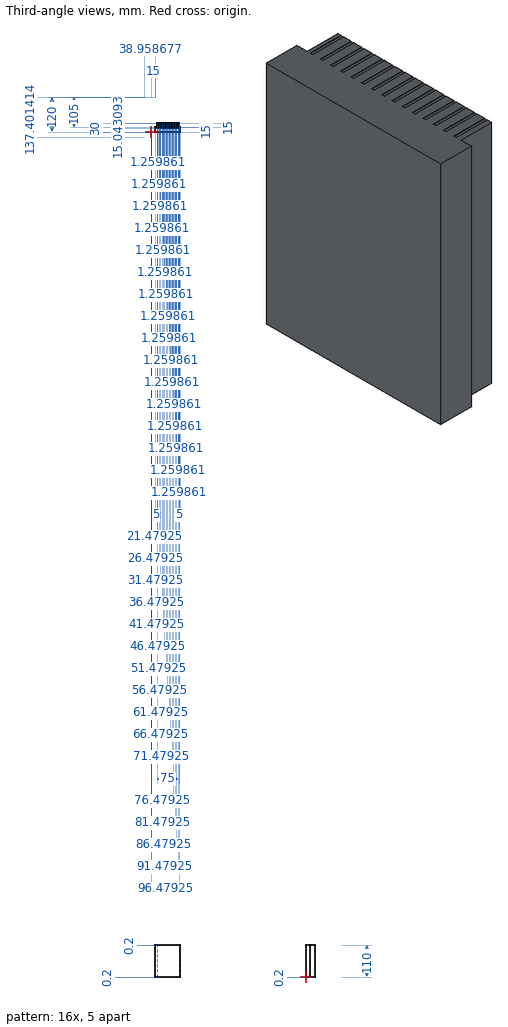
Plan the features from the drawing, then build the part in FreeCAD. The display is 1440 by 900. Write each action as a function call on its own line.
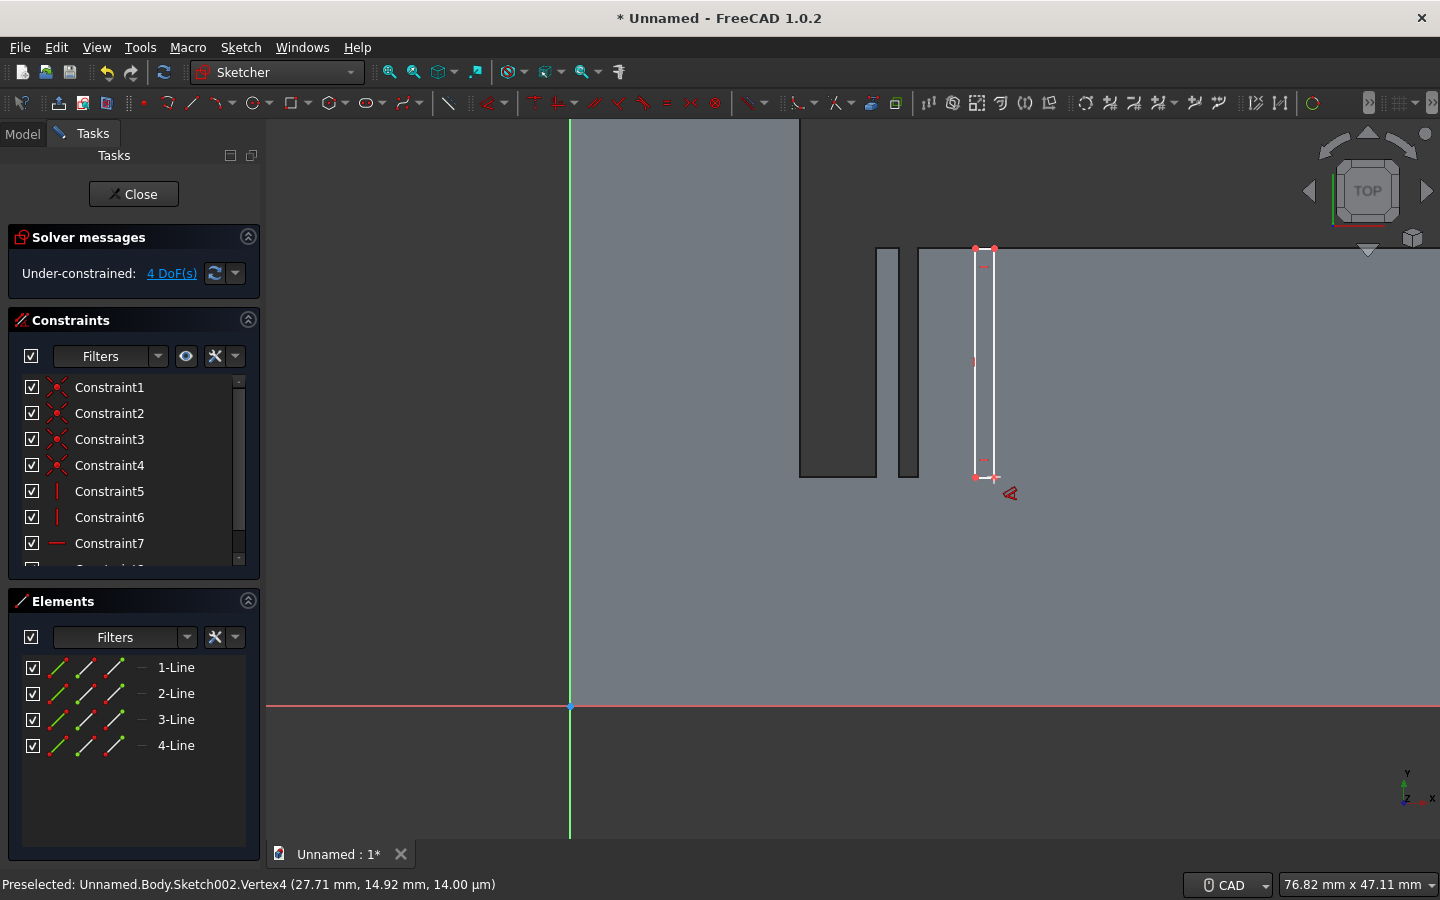
click(975, 249)
click(536, 478)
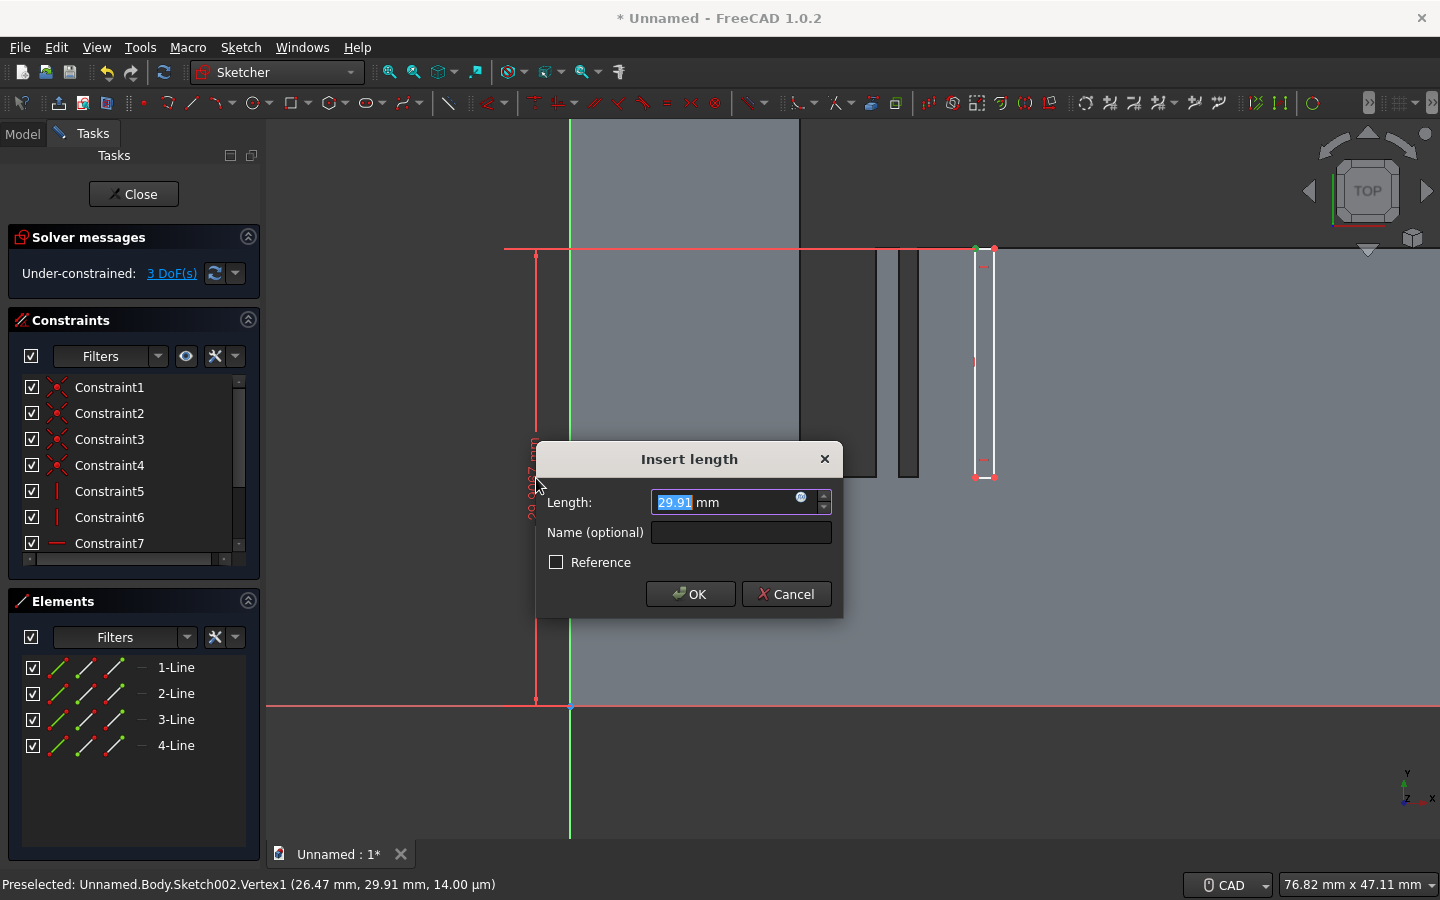
text(30)
key(Return)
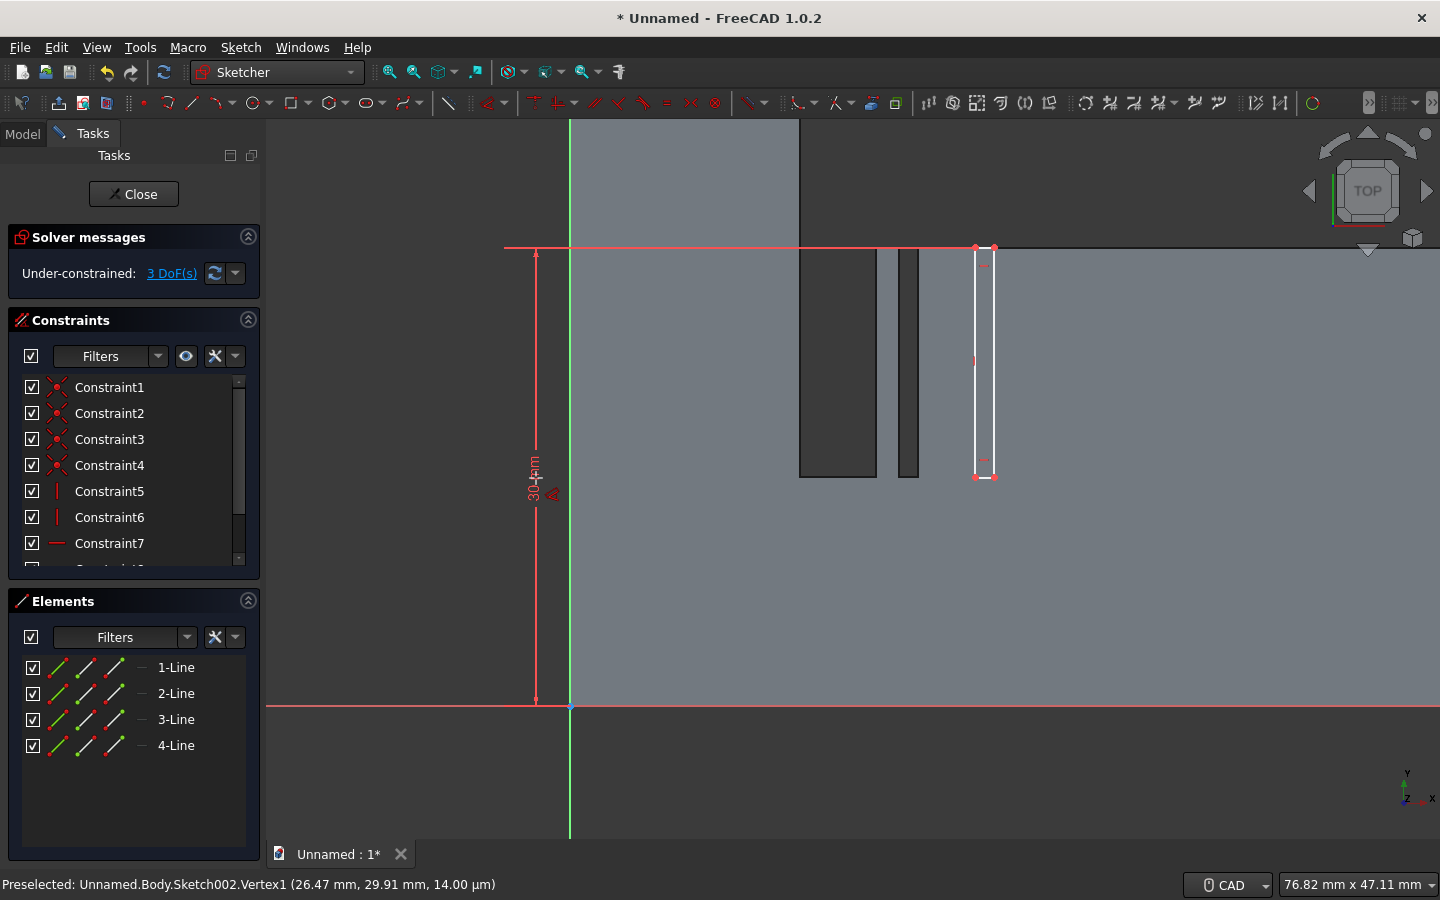
scroll(985, 478, up, 4)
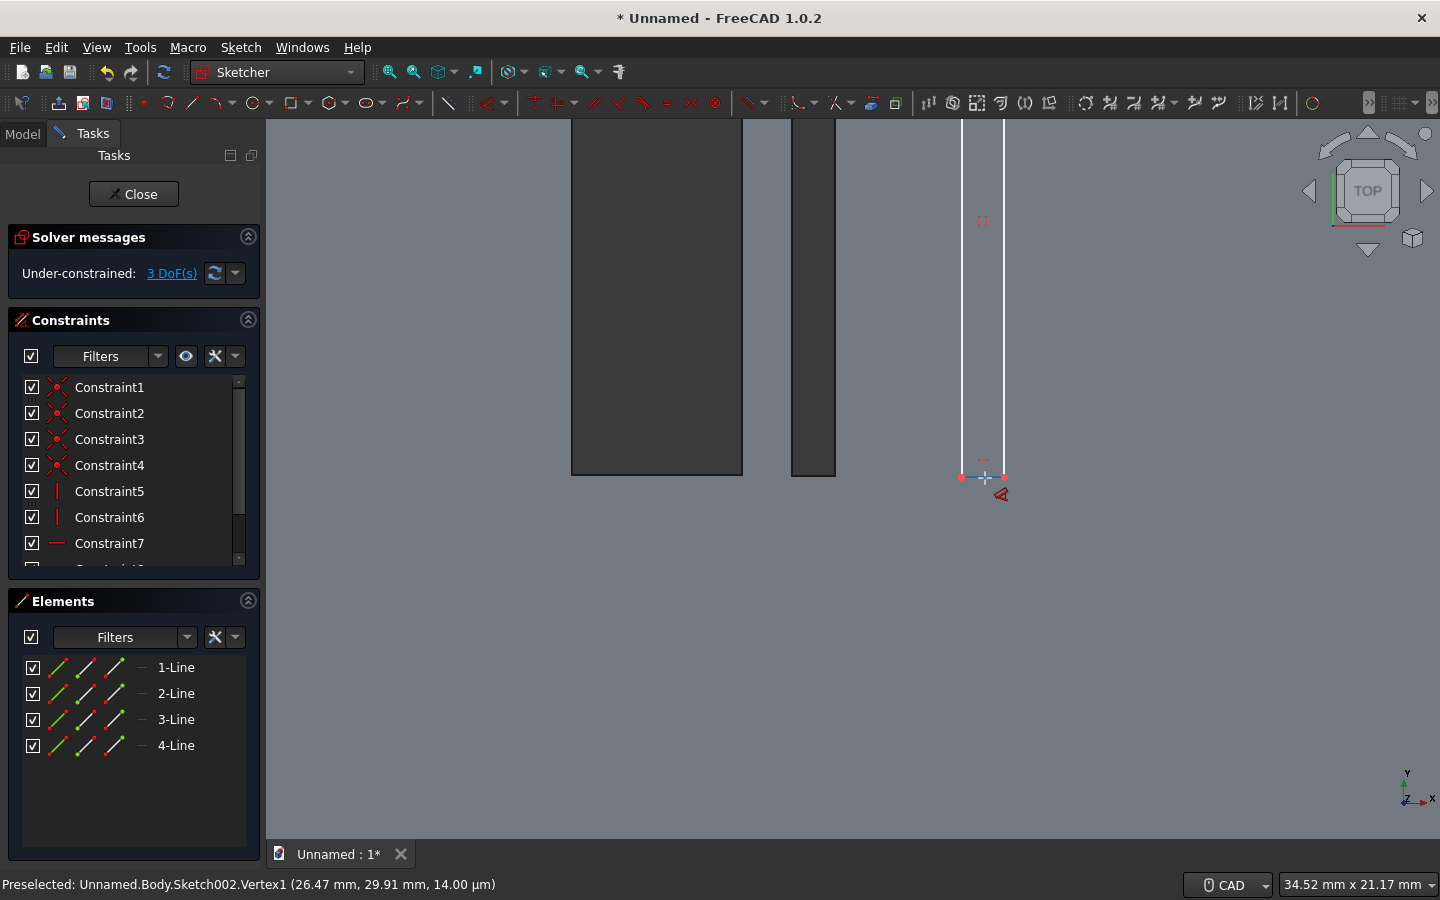
click(983, 477)
click(983, 511)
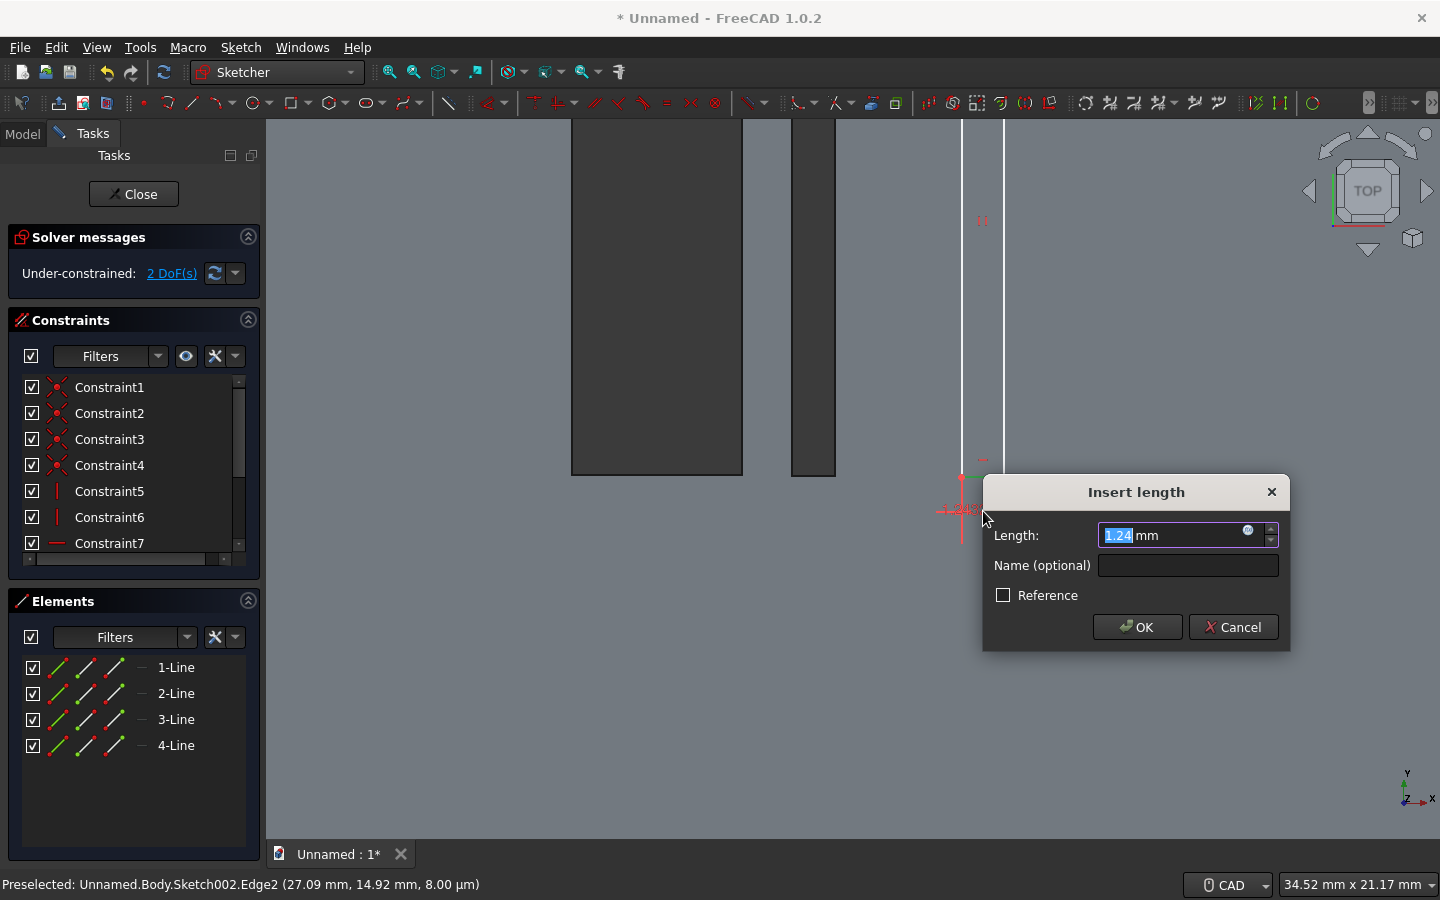
text(1.259861)
key(Return)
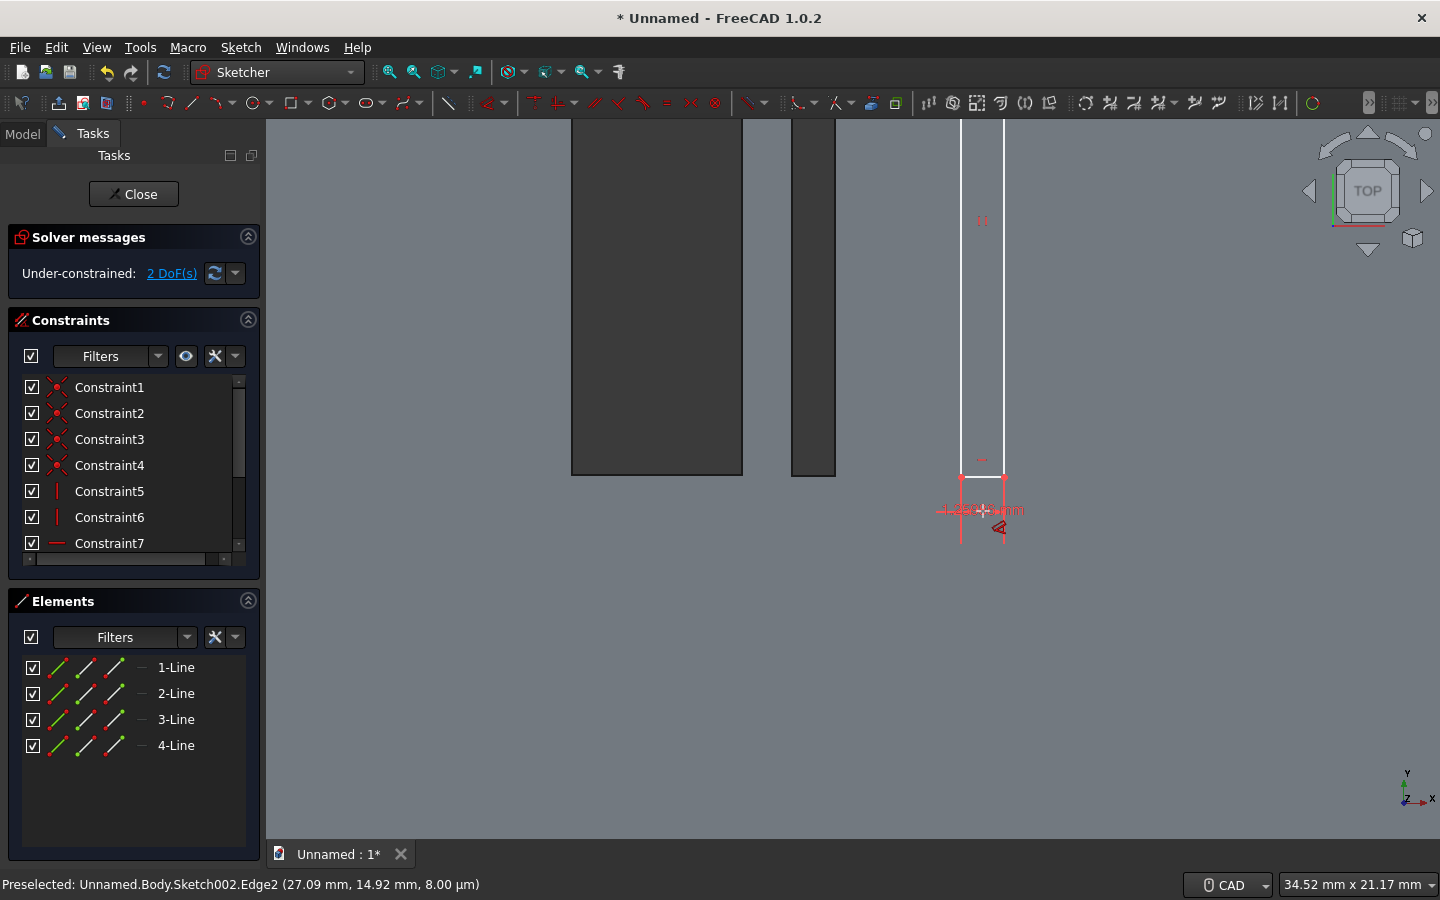
click(961, 324)
click(927, 312)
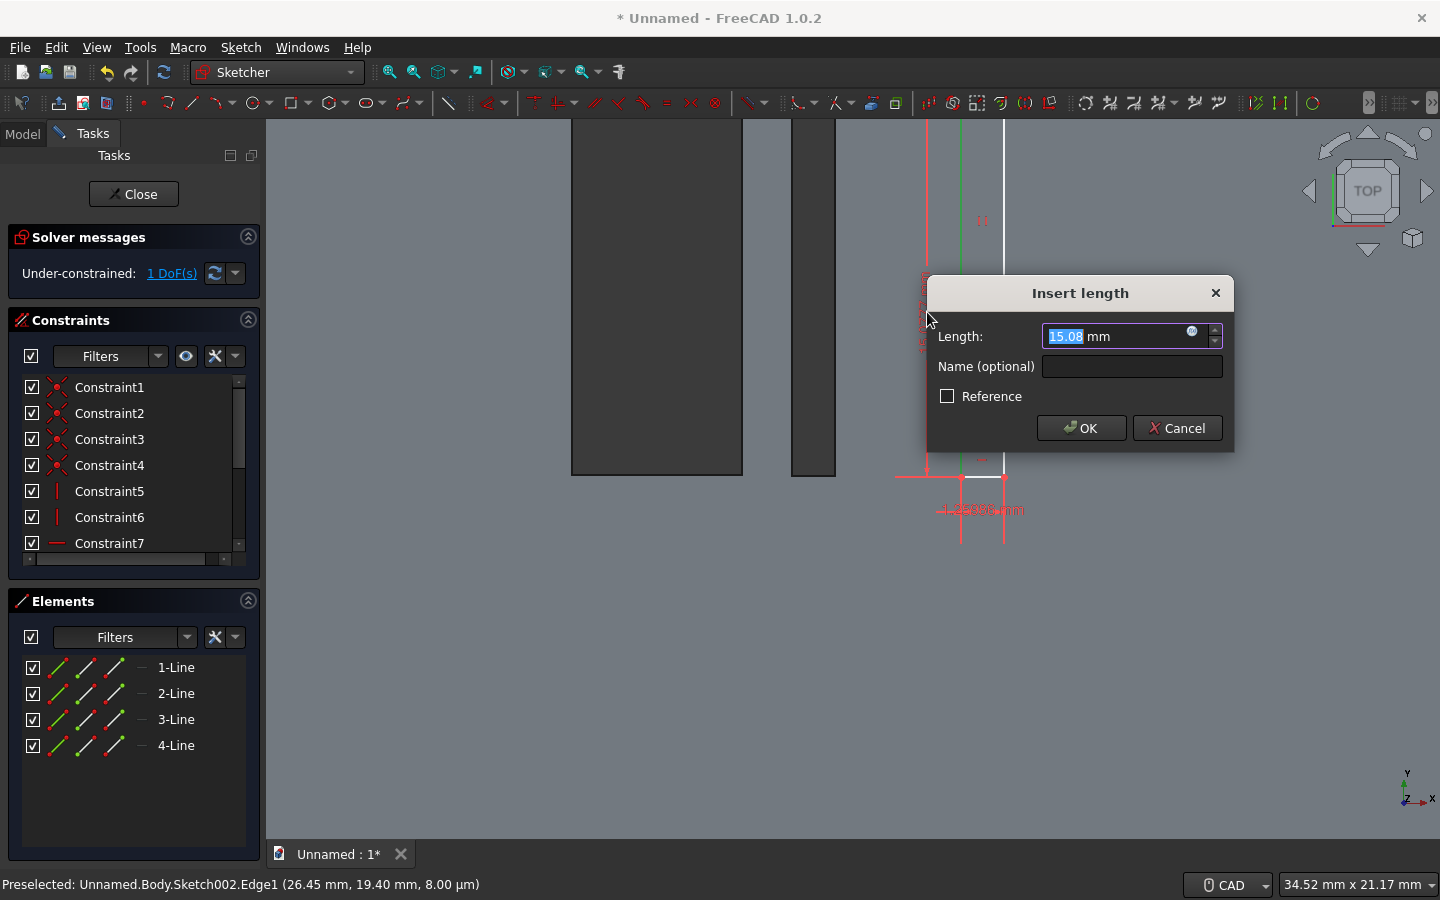
text(15.043093)
key(Return)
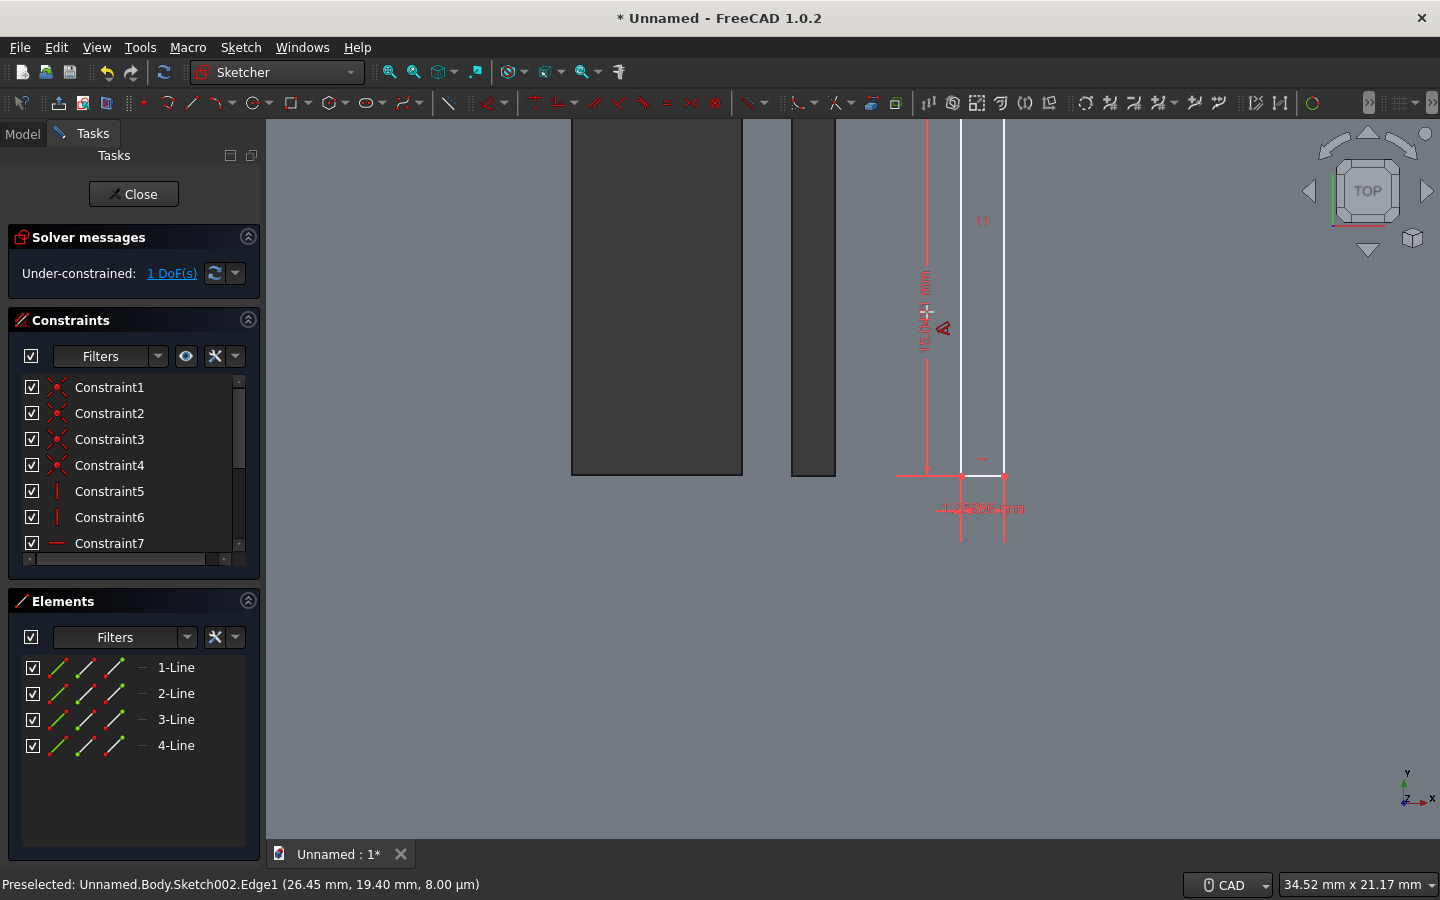
scroll(989, 482, down, 4)